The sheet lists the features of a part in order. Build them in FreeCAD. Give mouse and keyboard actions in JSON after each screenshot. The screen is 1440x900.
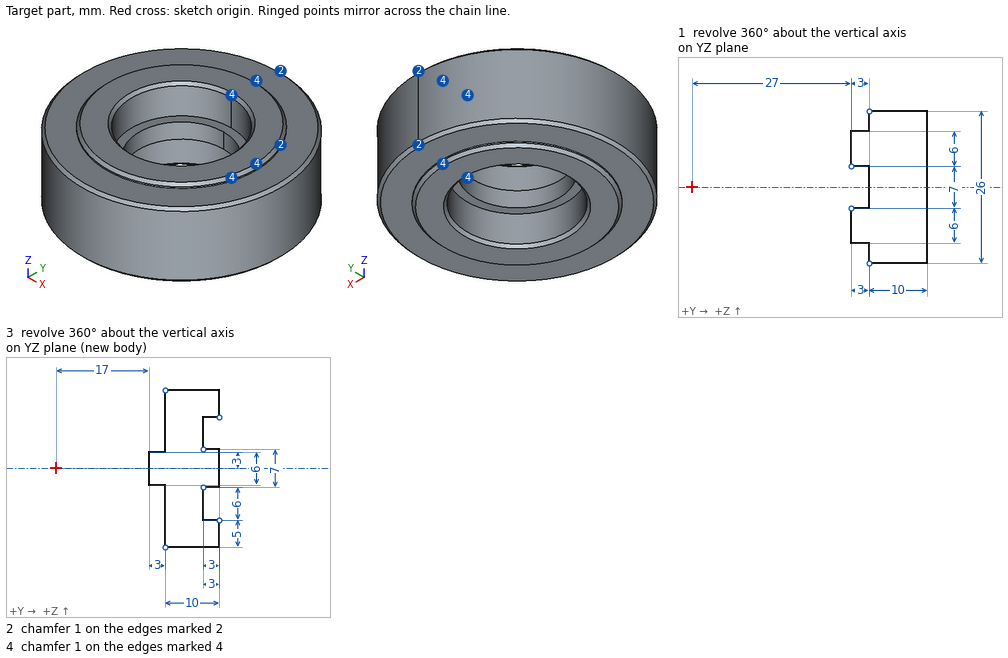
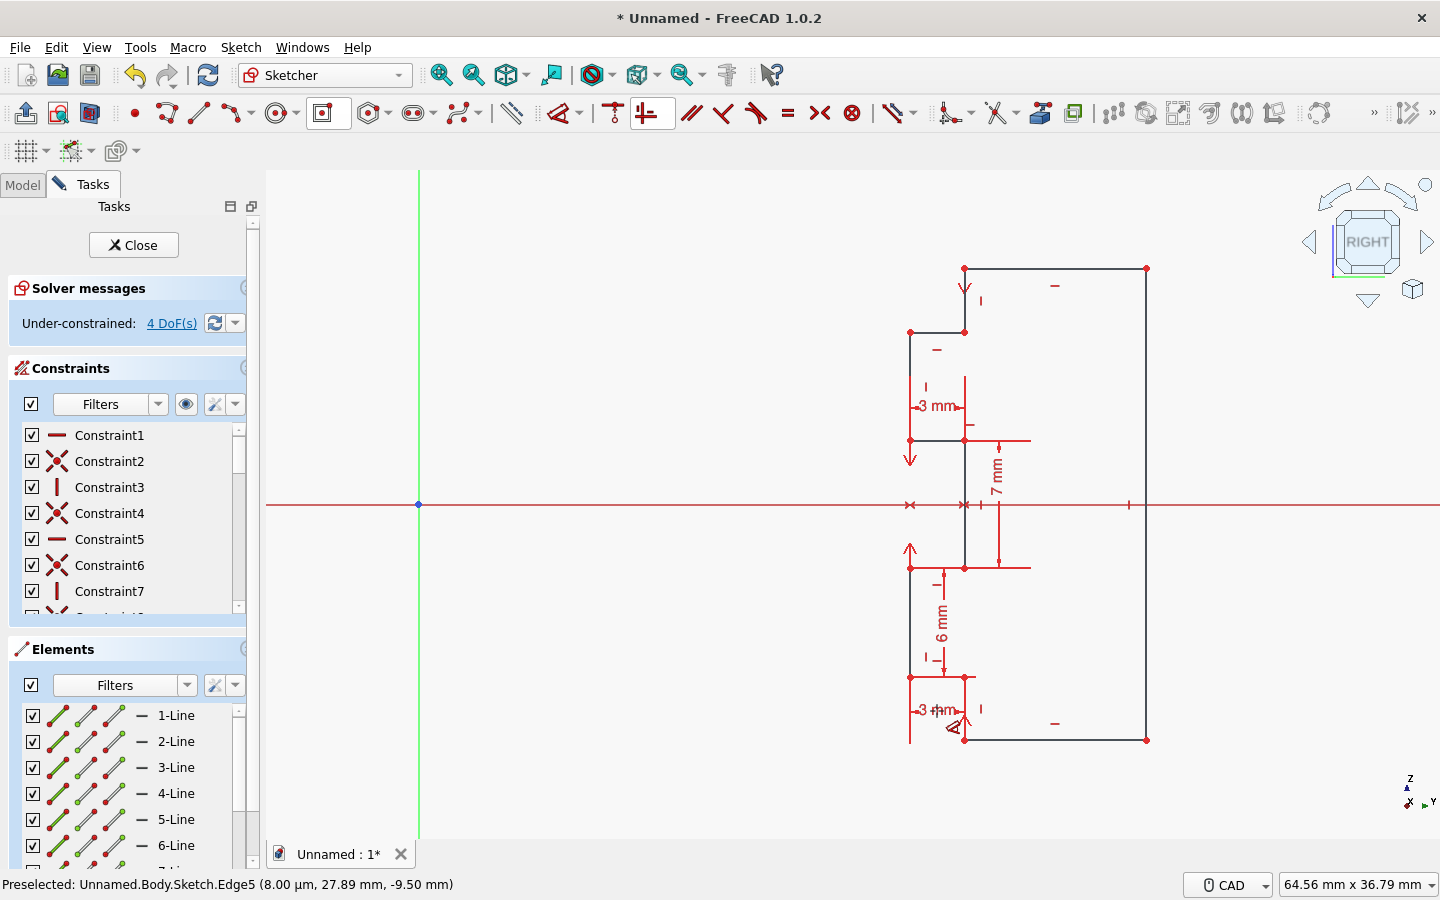
{"action": "left_click", "coordinate": [910, 365]}
{"action": "left_click", "coordinate": [944, 387]}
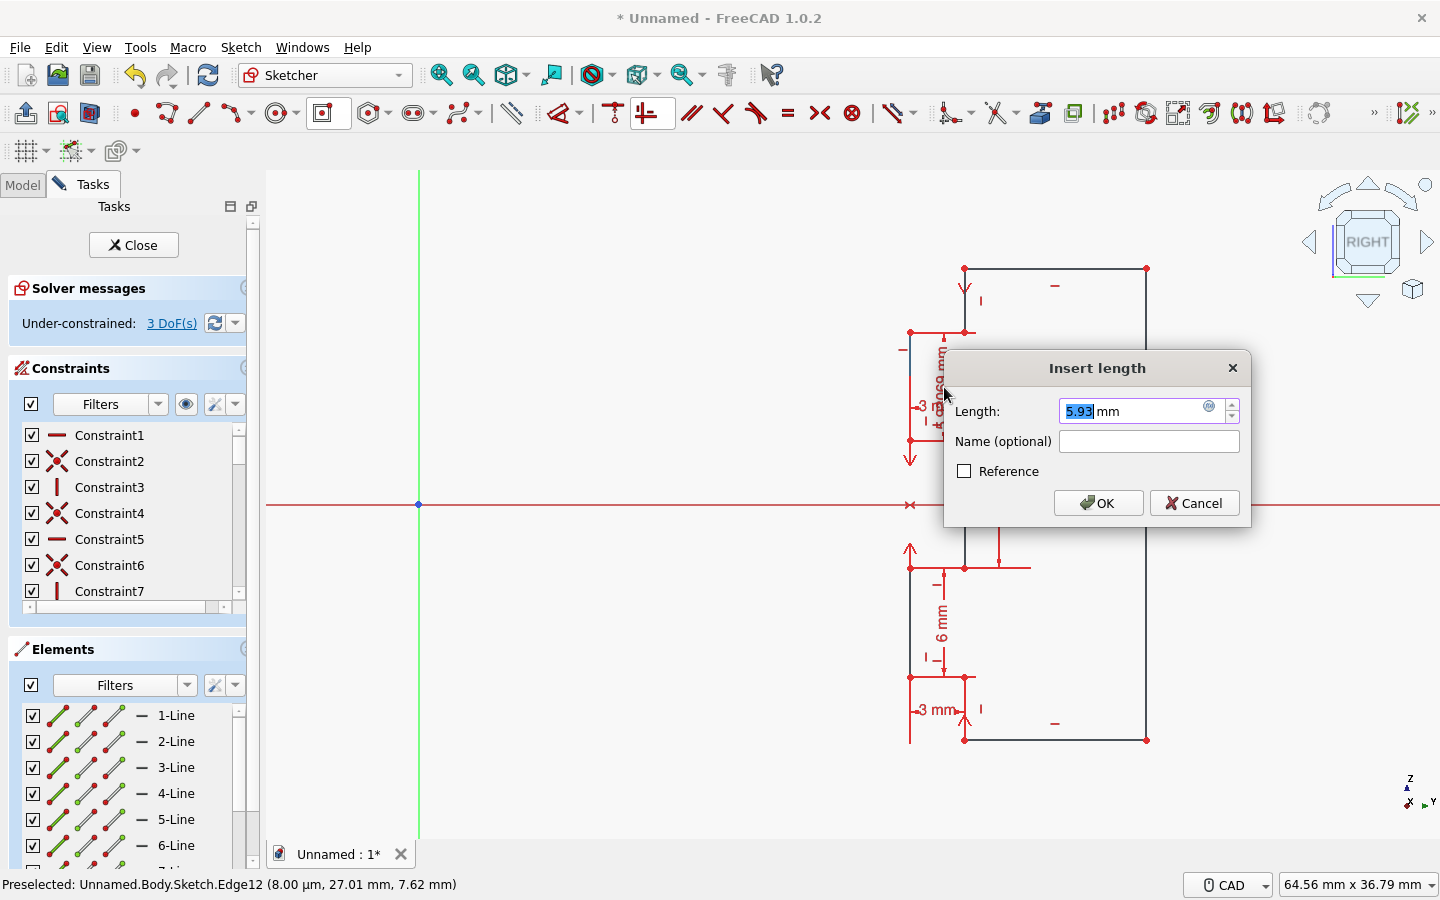
{"action": "type", "text": "6"}
{"action": "key", "text": "Return"}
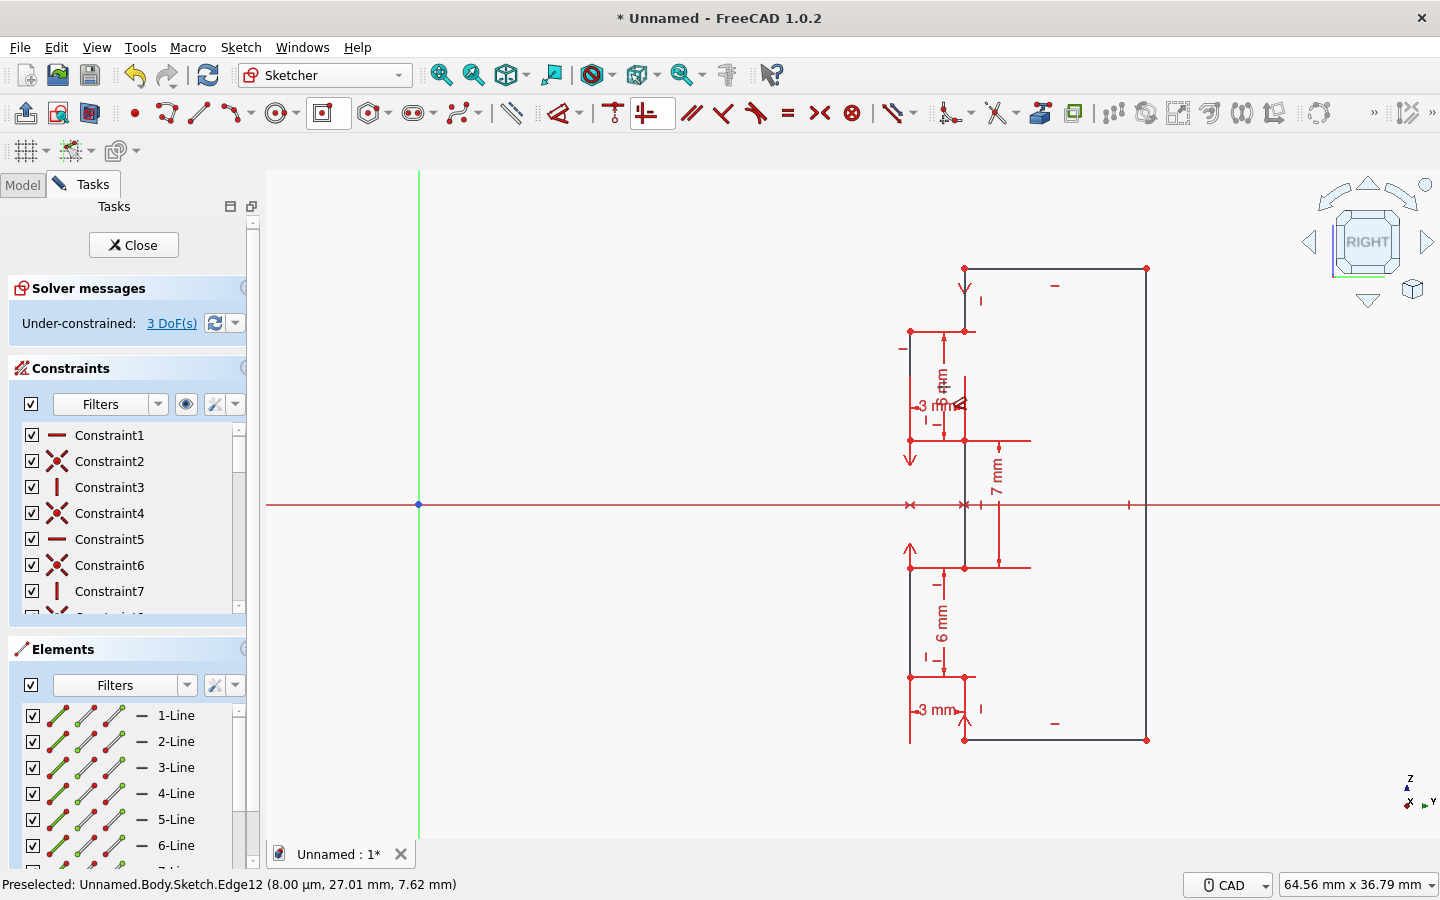
{"action": "left_click", "coordinate": [1019, 740]}
{"action": "left_click", "coordinate": [1055, 774]}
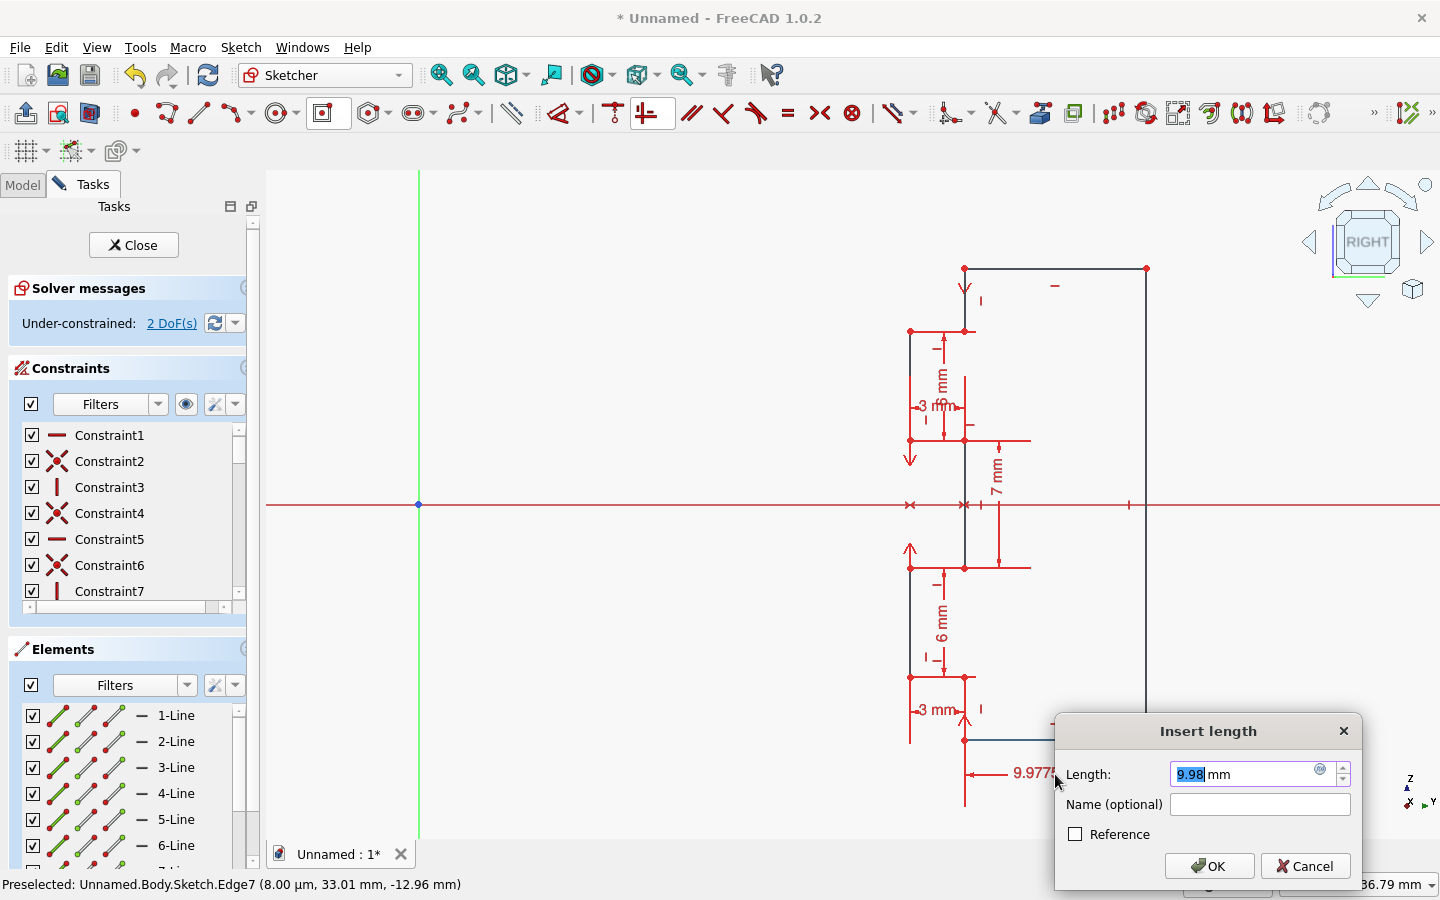
{"action": "type", "text": "10"}
{"action": "key", "text": "Return"}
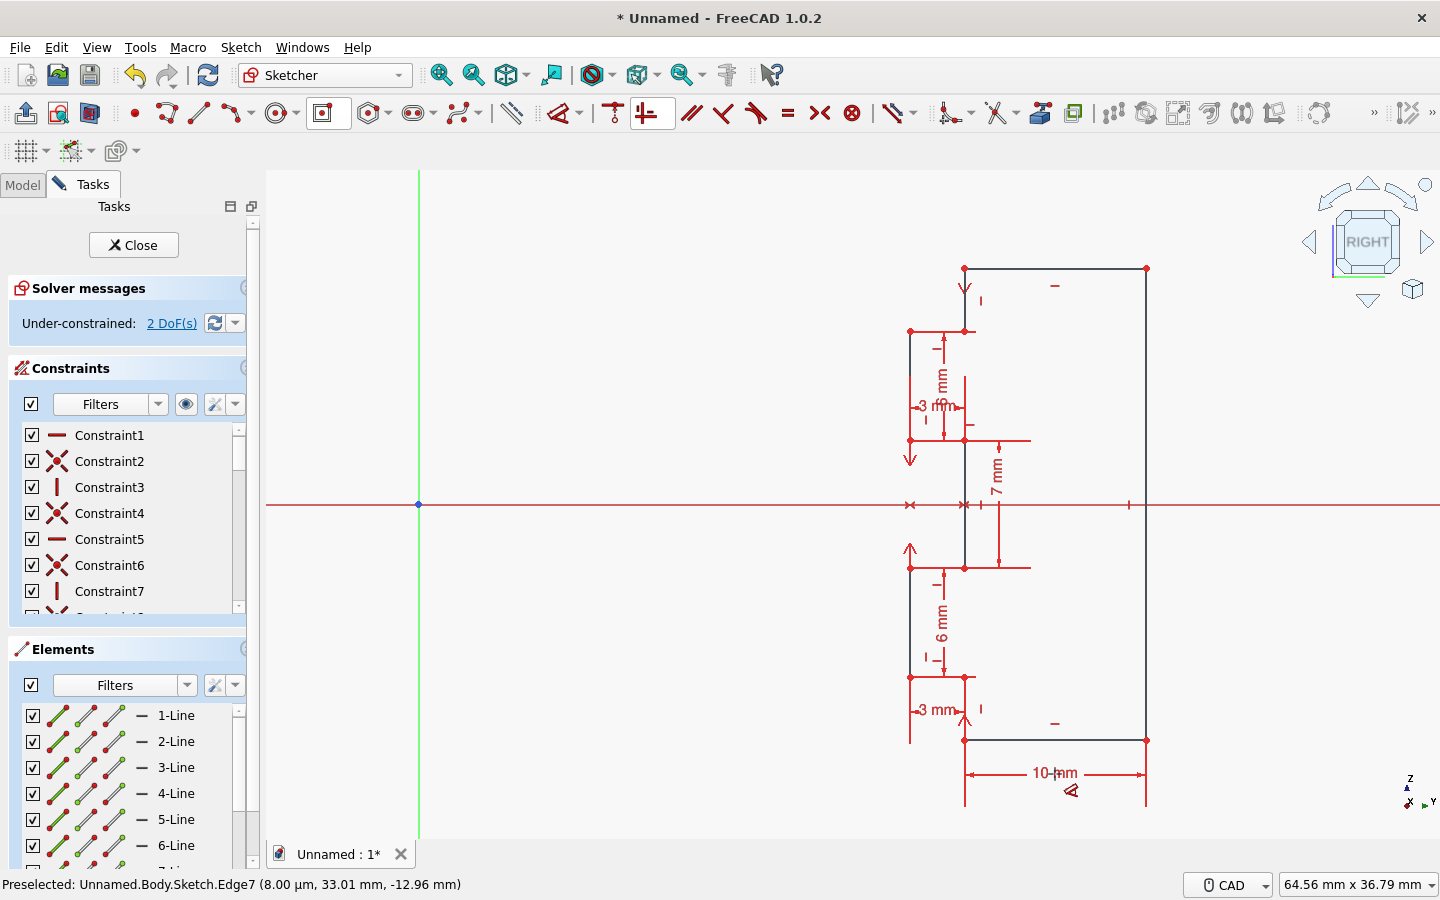
{"action": "left_click", "coordinate": [1146, 599]}
{"action": "left_click", "coordinate": [1180, 396]}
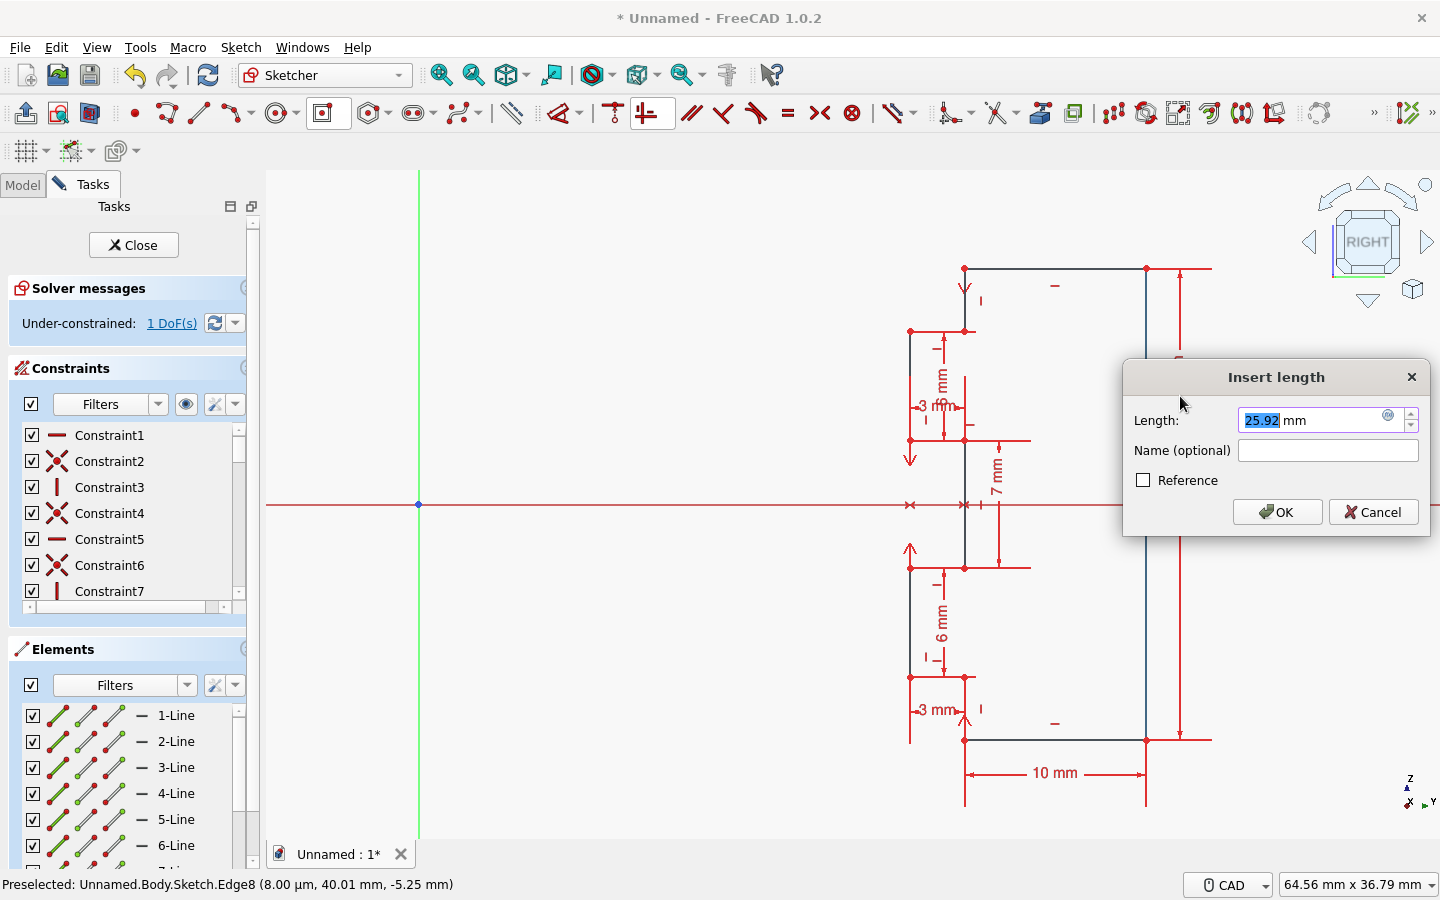
{"action": "type", "text": "26"}
{"action": "key", "text": "Return"}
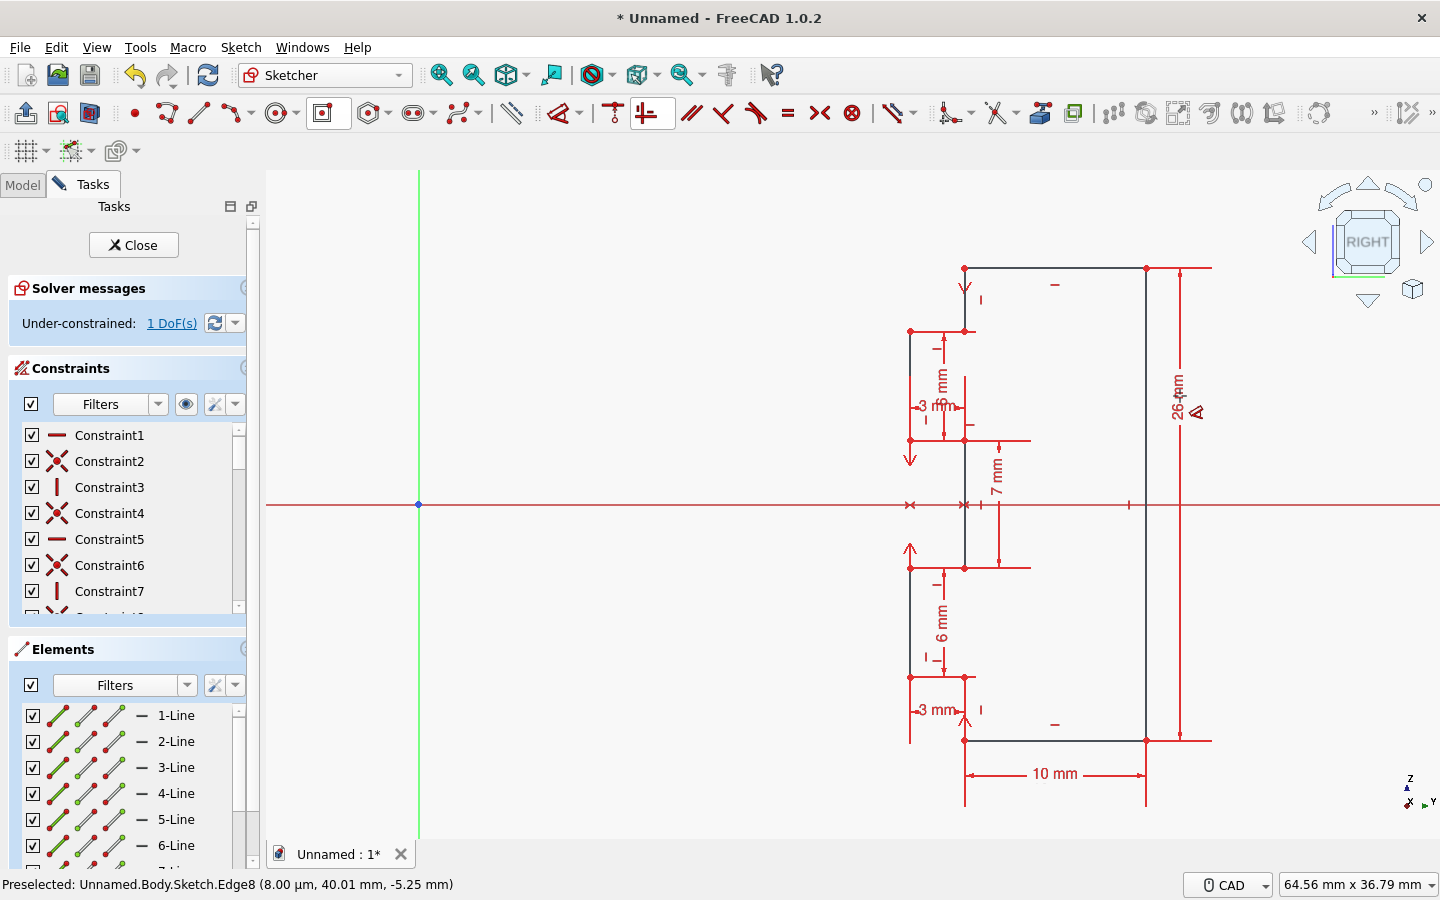
{"action": "left_click", "coordinate": [910, 441]}
{"action": "left_click", "coordinate": [664, 407]}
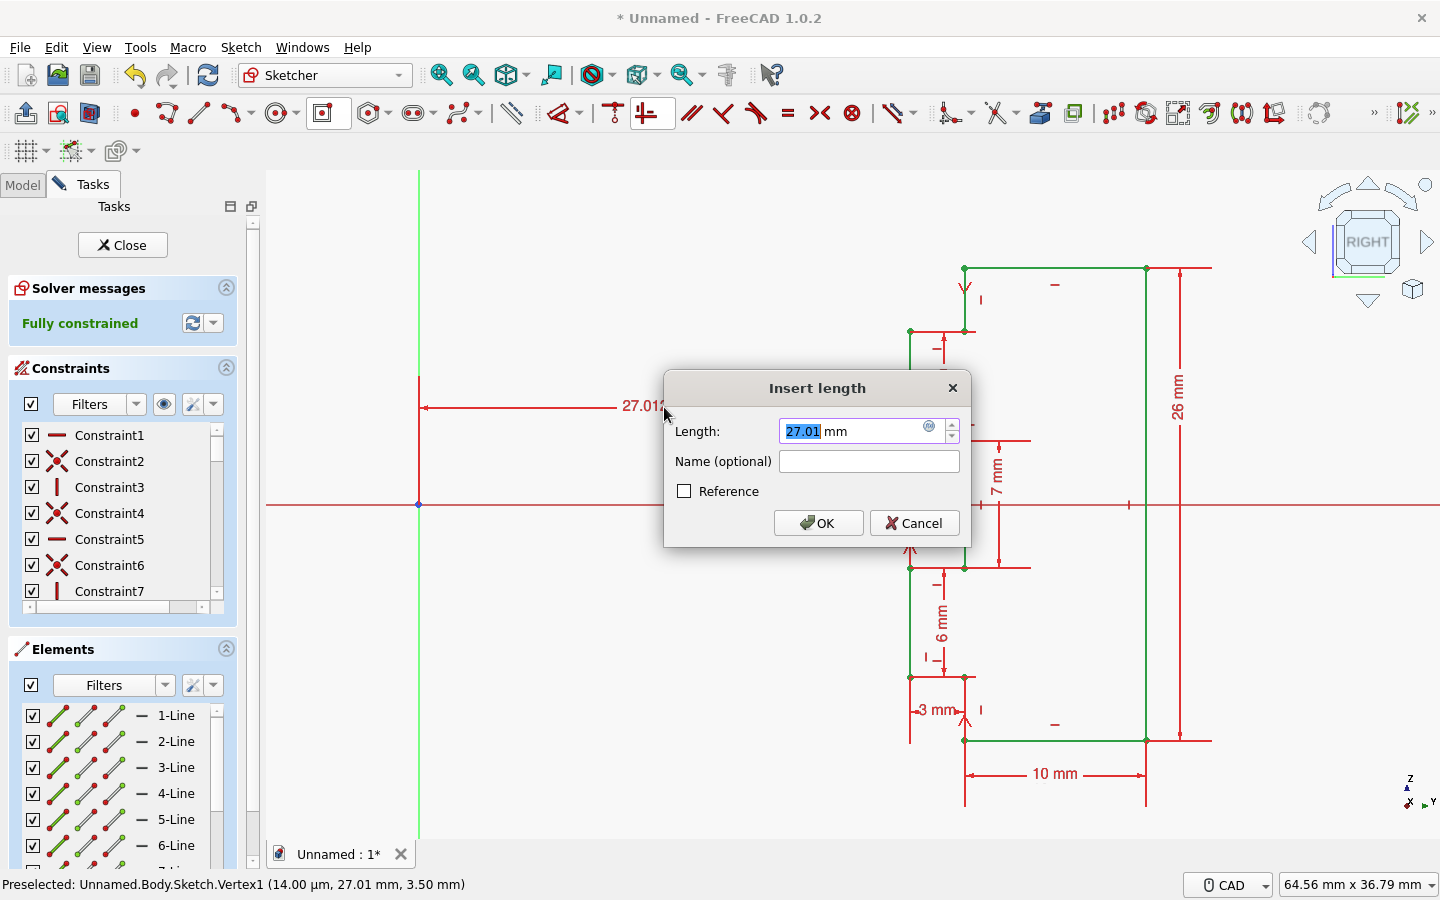
{"action": "type", "text": "27"}
{"action": "key", "text": "Return"}
{"action": "key", "text": "Escape"}